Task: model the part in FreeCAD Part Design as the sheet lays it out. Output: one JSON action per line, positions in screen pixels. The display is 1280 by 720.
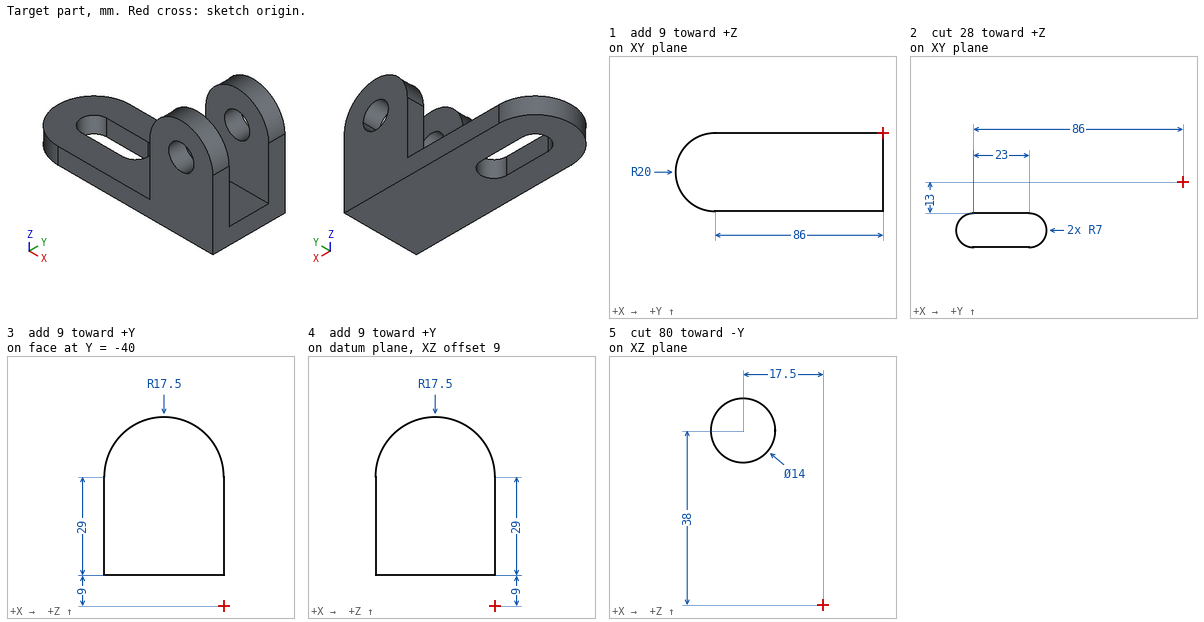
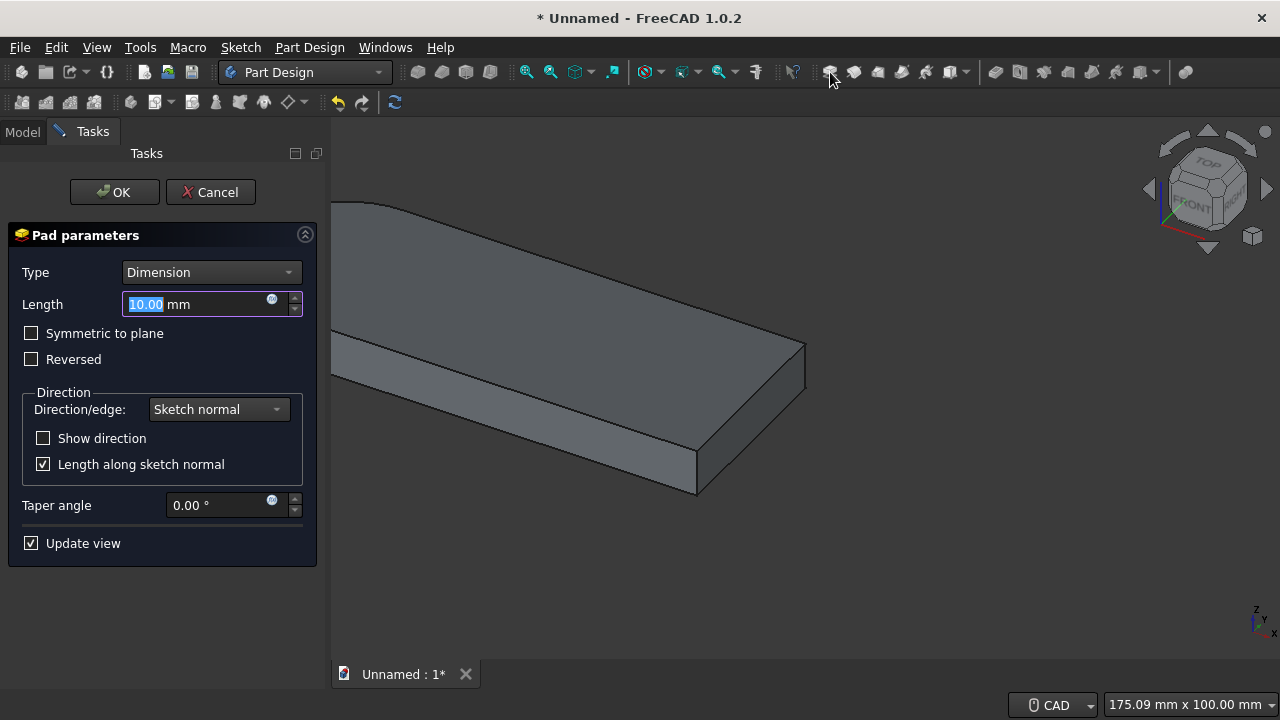
{"action": "type", "text": "9"}
{"action": "key", "text": "Tab"}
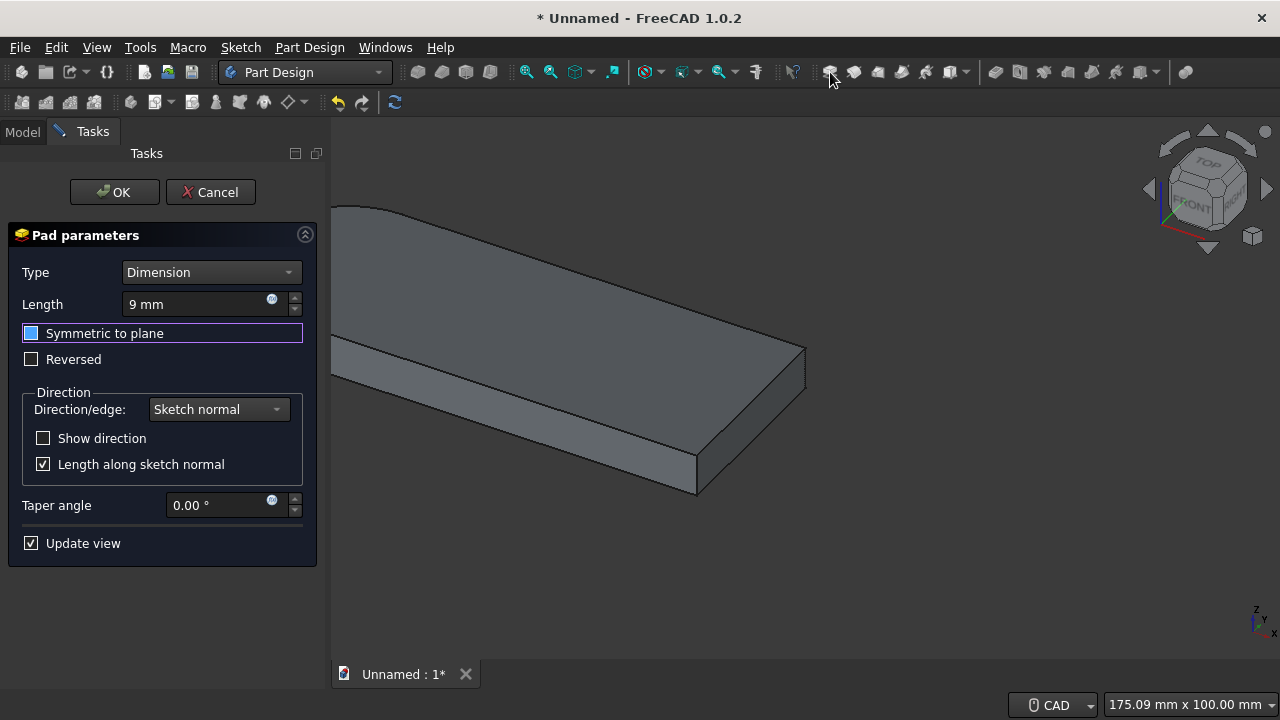
{"action": "left_click", "coordinate": [115, 192]}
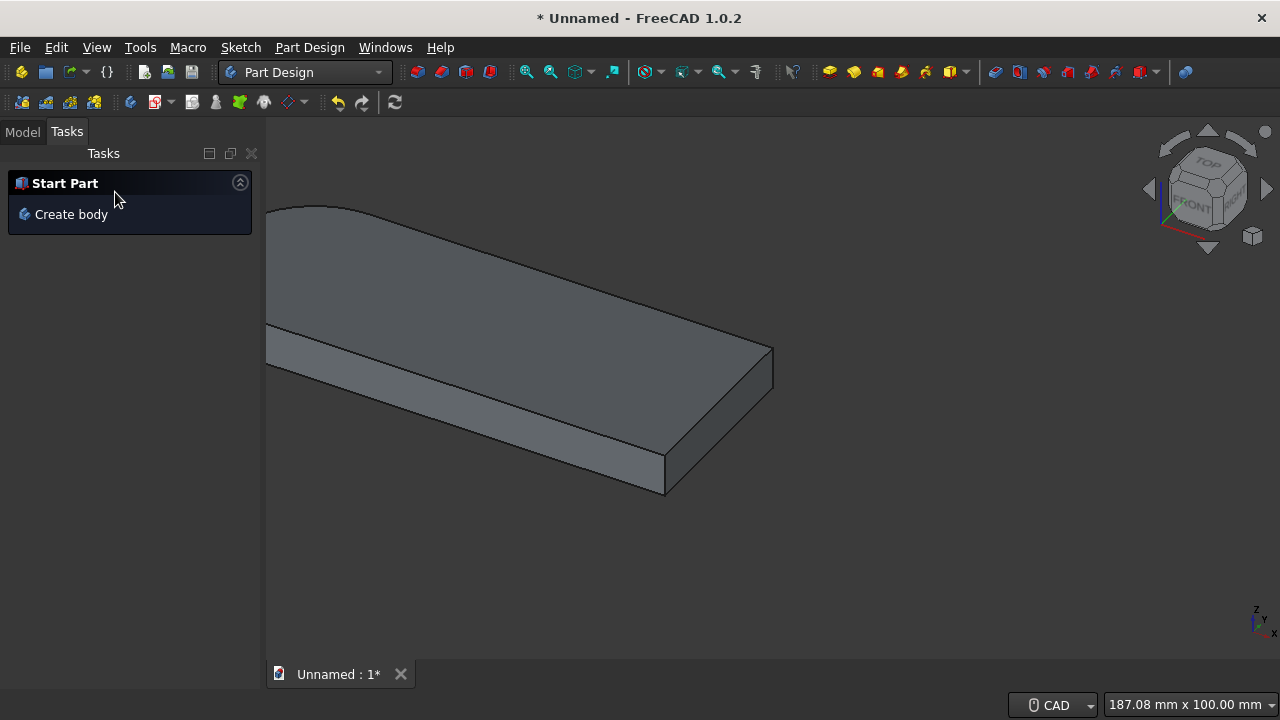
{"action": "left_click", "coordinate": [528, 72]}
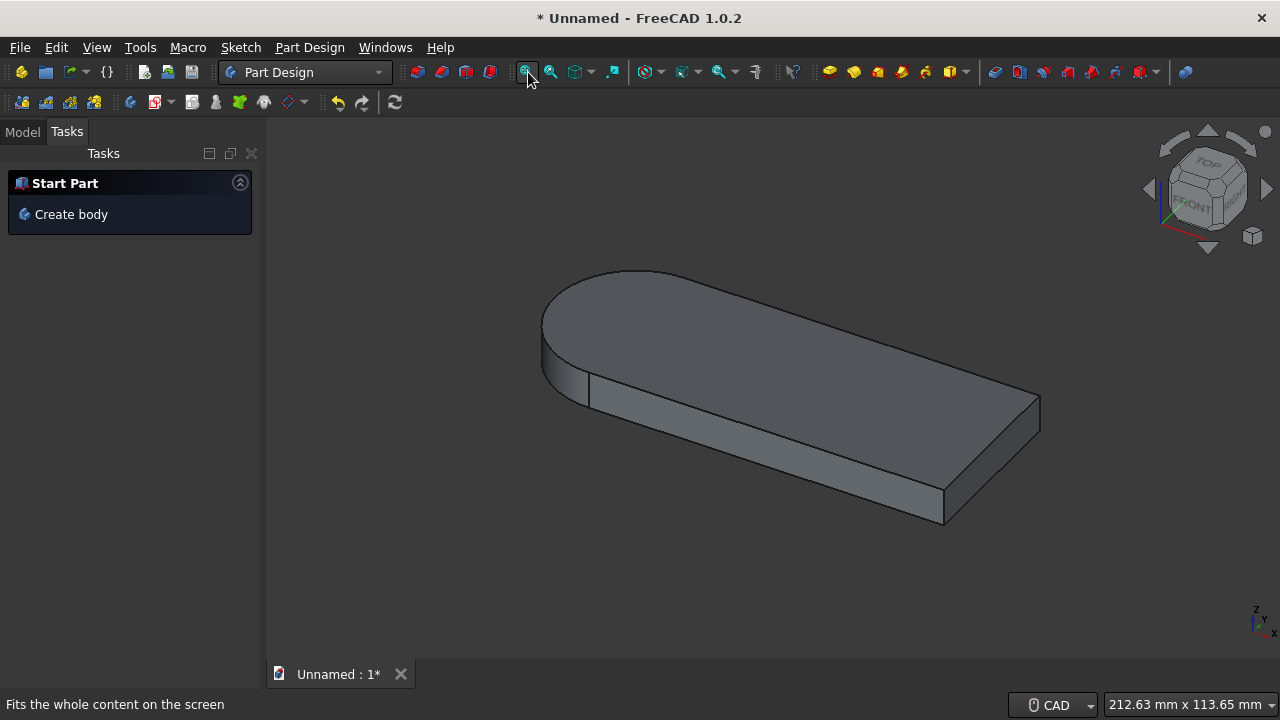
{"action": "left_click", "coordinate": [156, 102]}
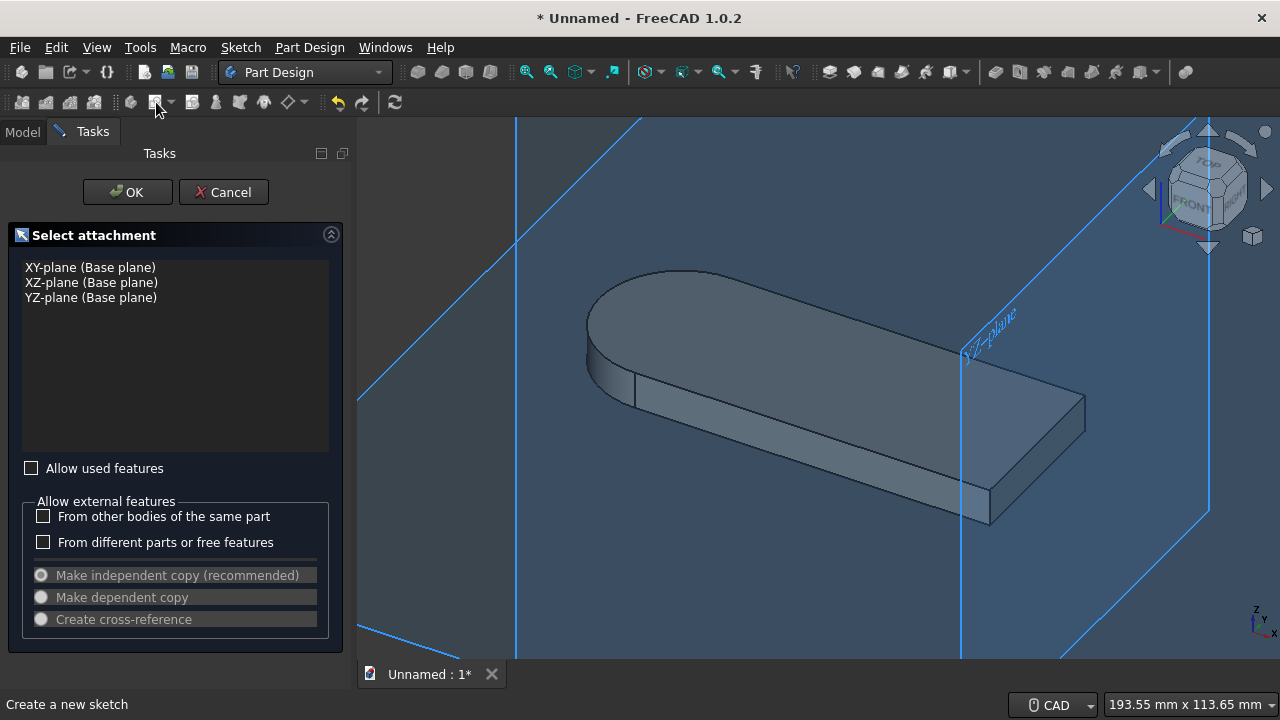
{"action": "left_click", "coordinate": [82, 268]}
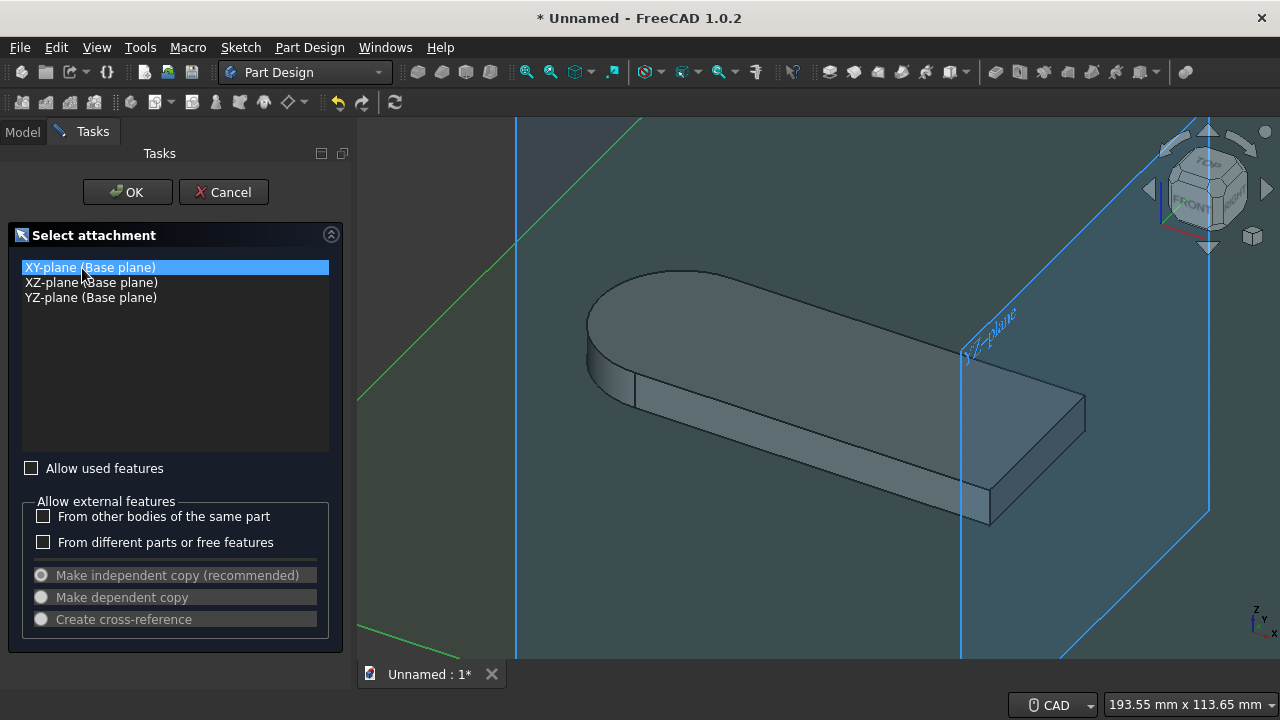
{"action": "left_click", "coordinate": [128, 192]}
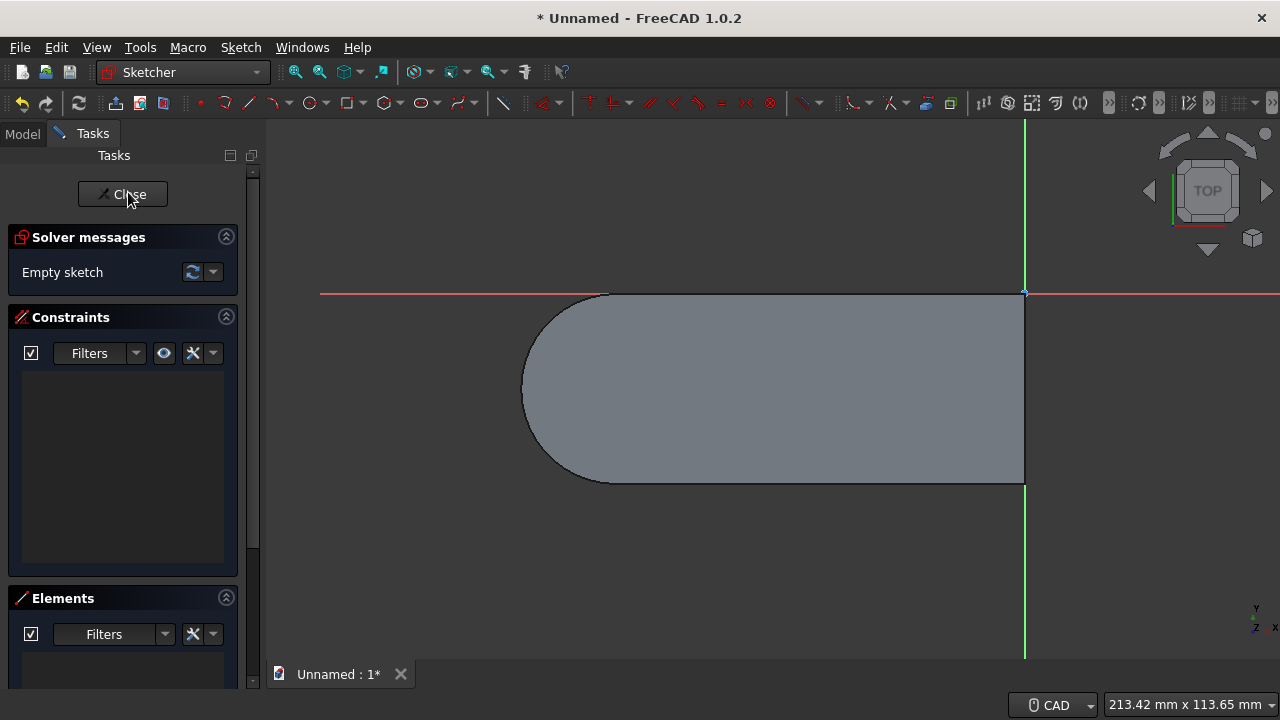
{"action": "left_click", "coordinate": [164, 104]}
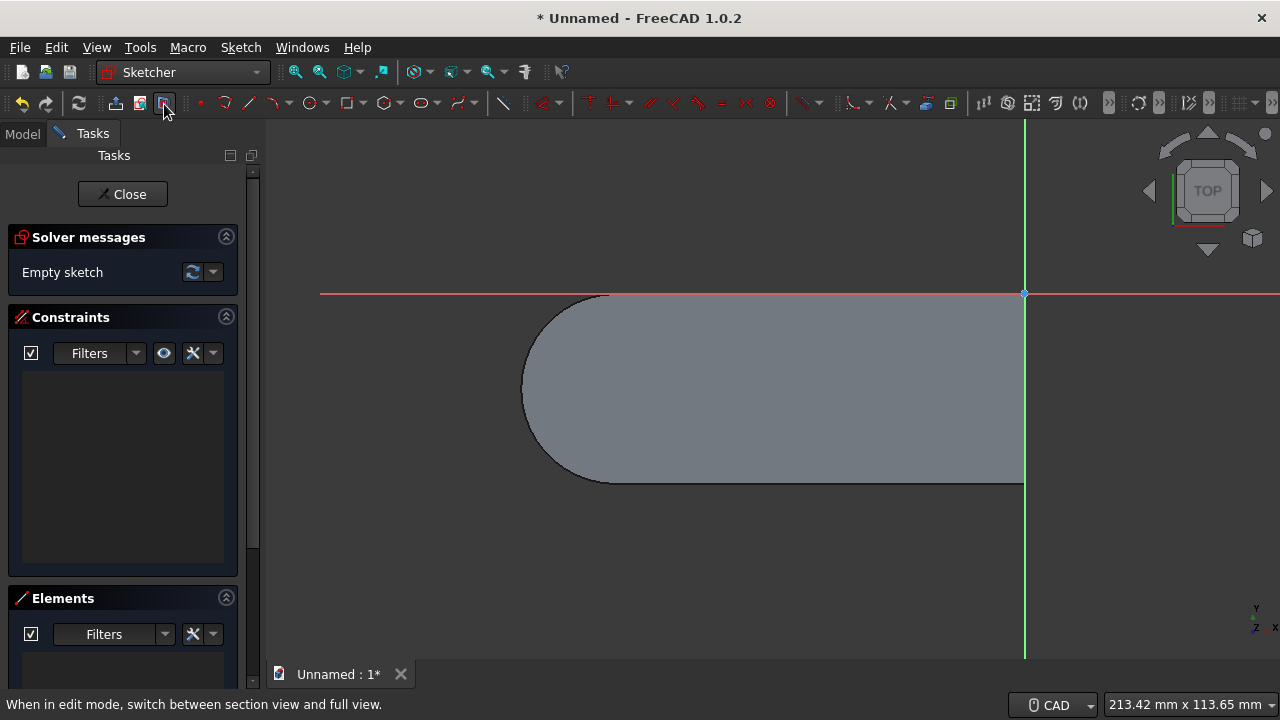
{"action": "scroll", "coordinate": [656, 389], "scroll_direction": "up", "scroll_amount": 6}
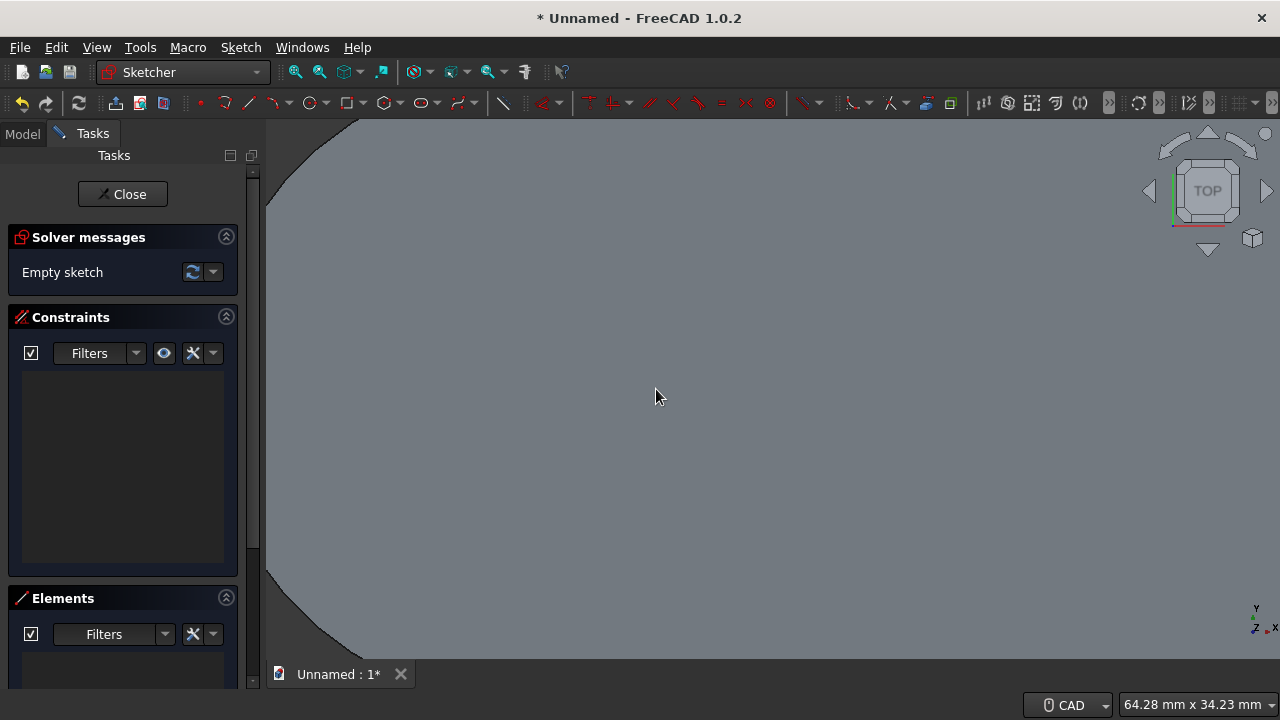
{"action": "left_click", "coordinate": [422, 104]}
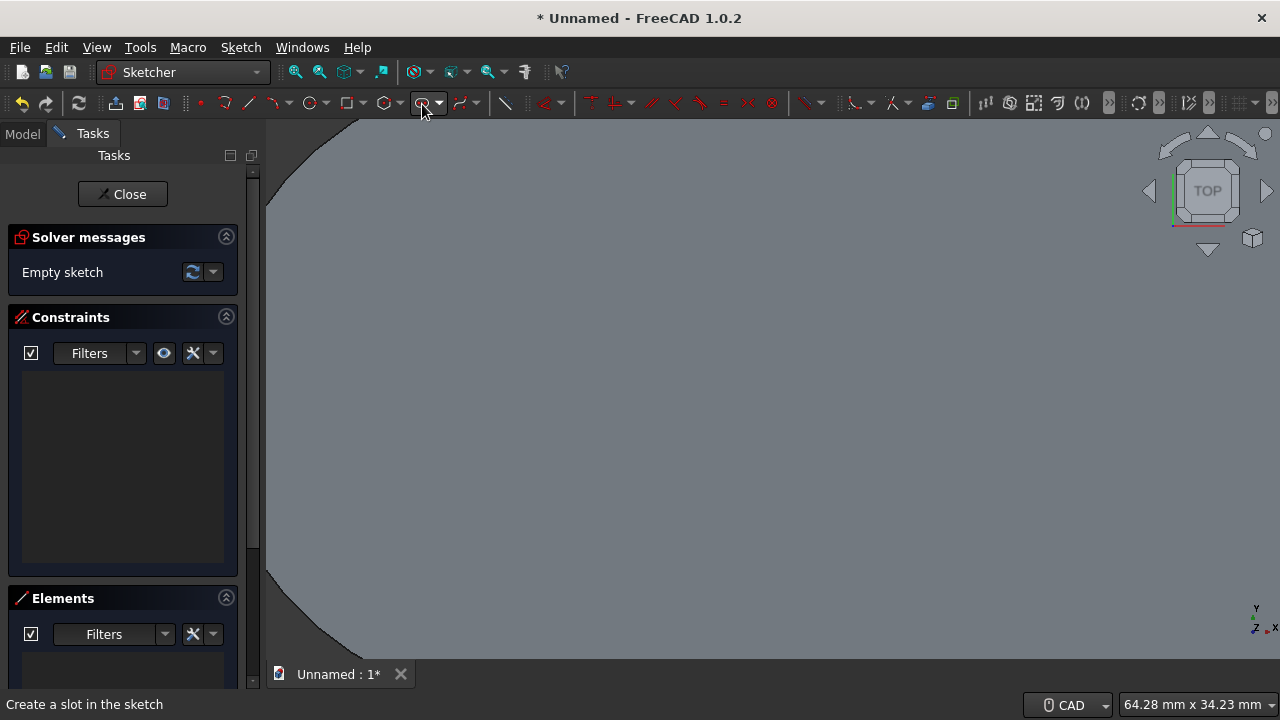
{"action": "left_click", "coordinate": [523, 388]}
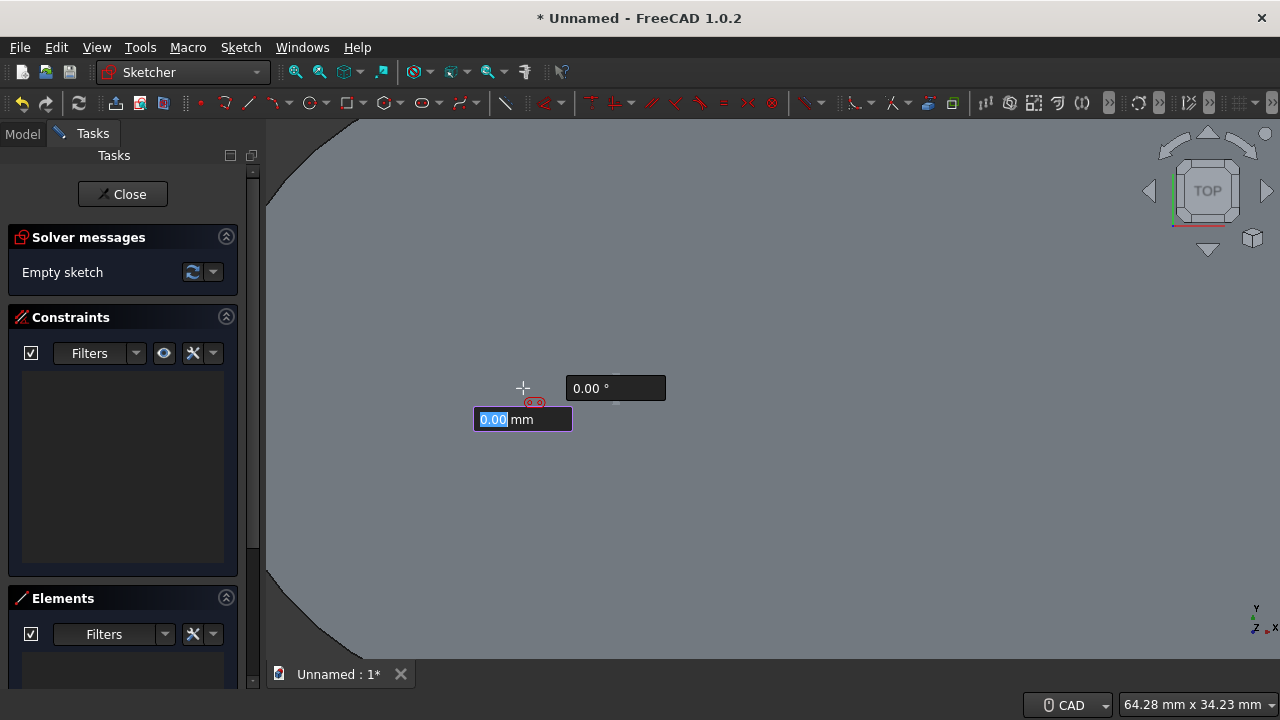
{"action": "left_click", "coordinate": [886, 388]}